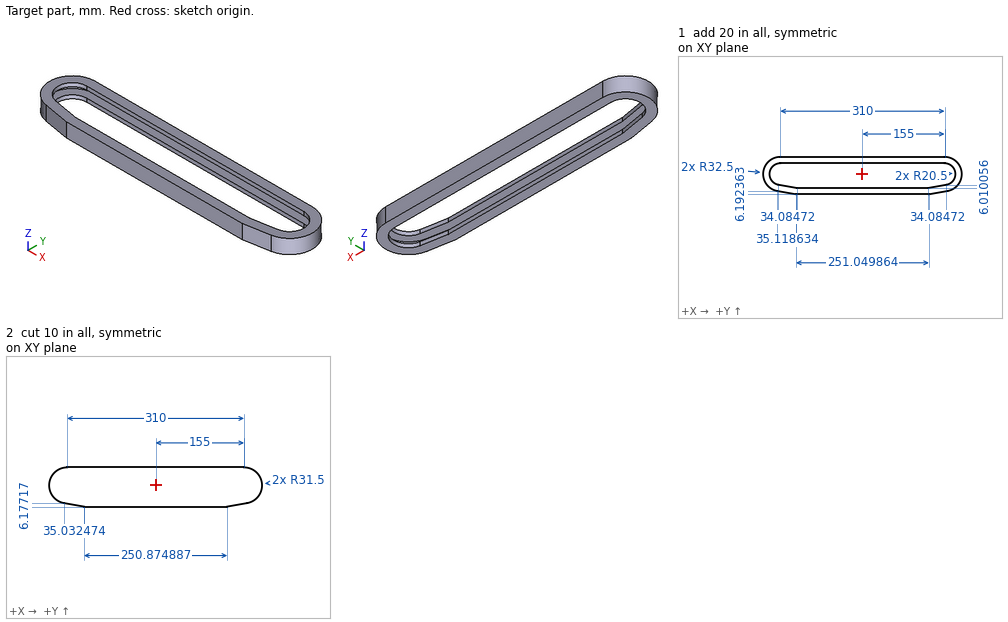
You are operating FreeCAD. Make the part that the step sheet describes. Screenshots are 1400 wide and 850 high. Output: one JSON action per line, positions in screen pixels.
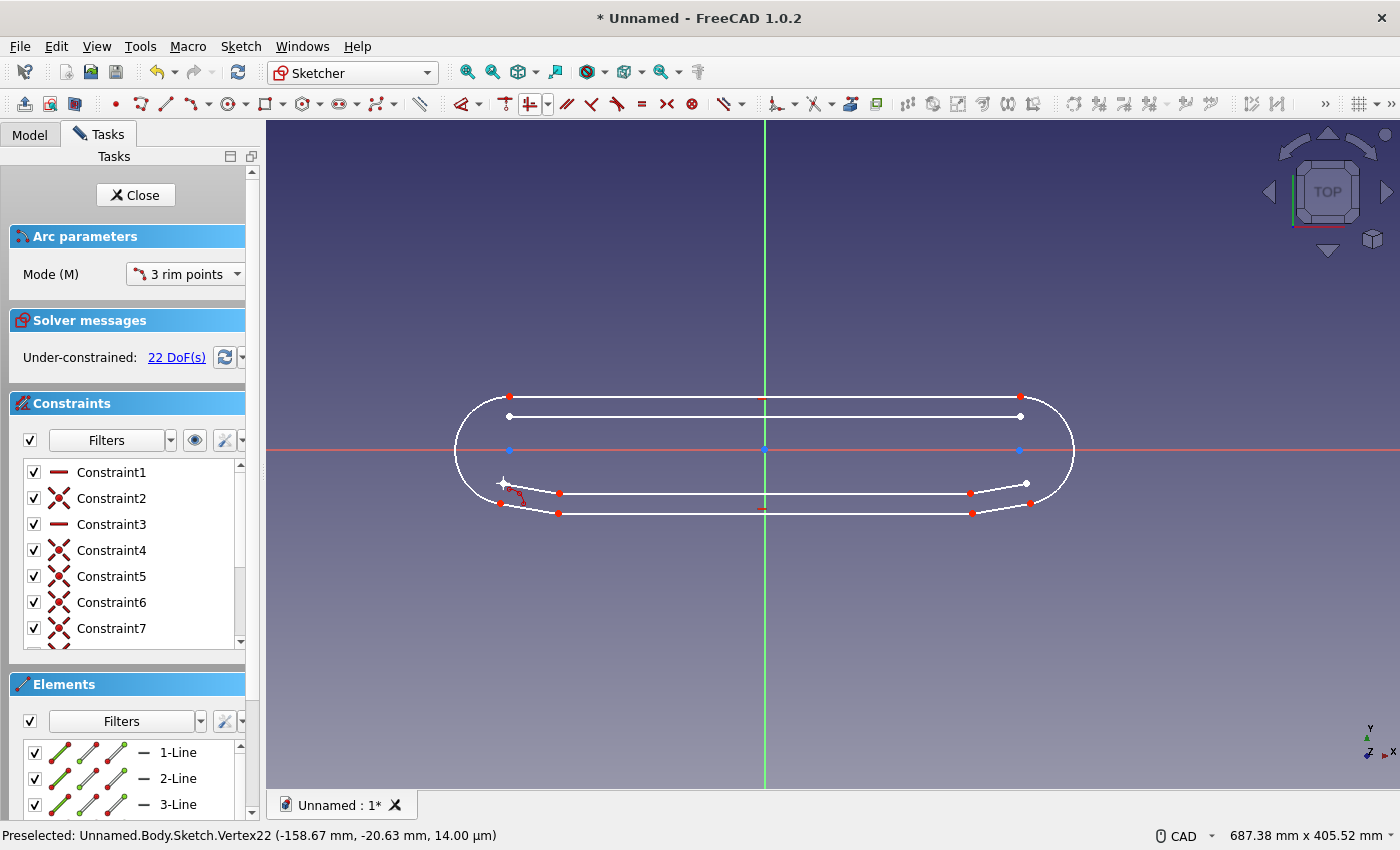
{"action": "left_click", "coordinate": [1020, 417]}
{"action": "left_click", "coordinate": [1026, 484]}
{"action": "left_click", "coordinate": [1050, 466]}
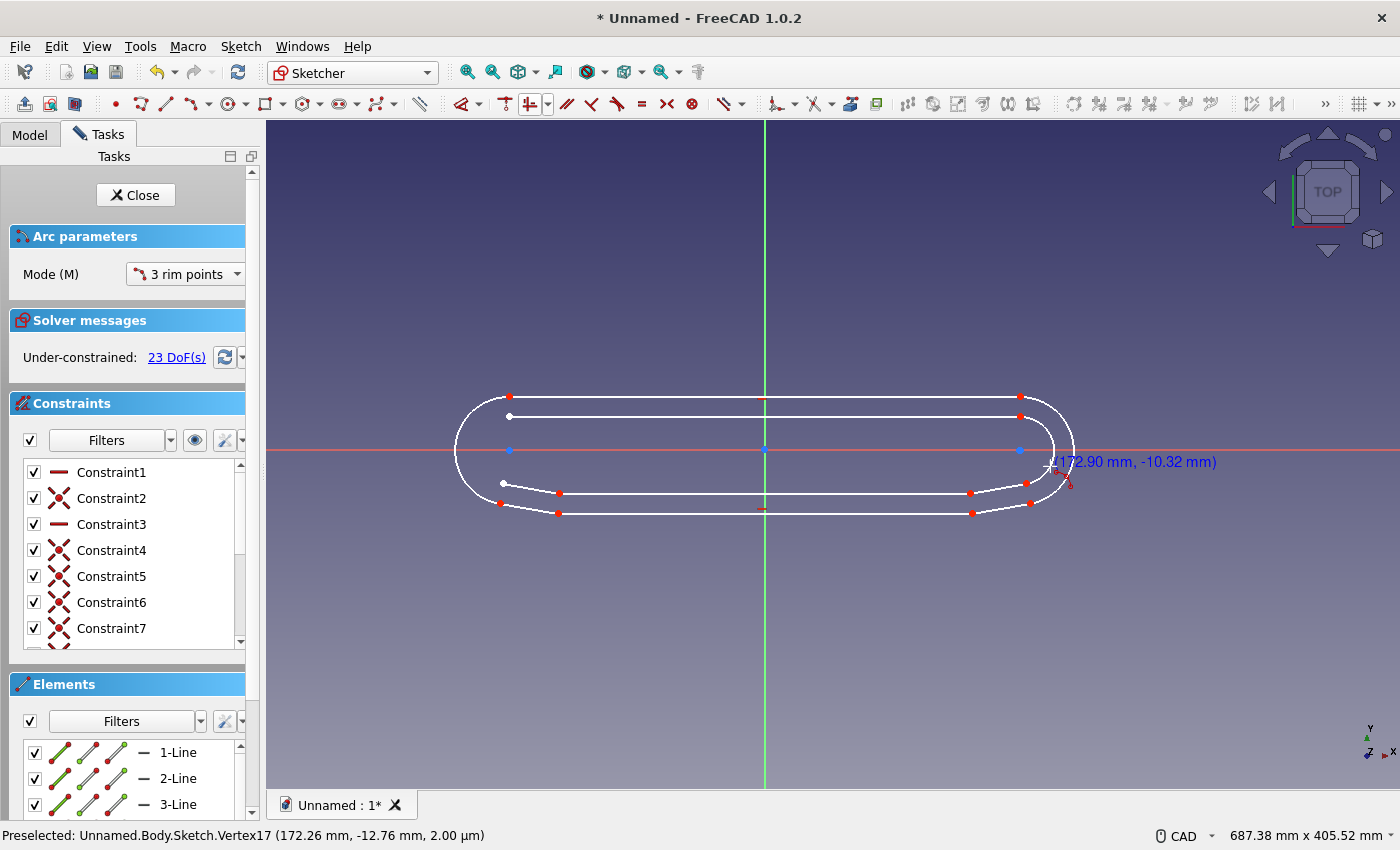
{"action": "left_click", "coordinate": [503, 484]}
{"action": "left_click", "coordinate": [509, 417]}
{"action": "left_click", "coordinate": [483, 429]}
{"action": "key", "text": "Escape"}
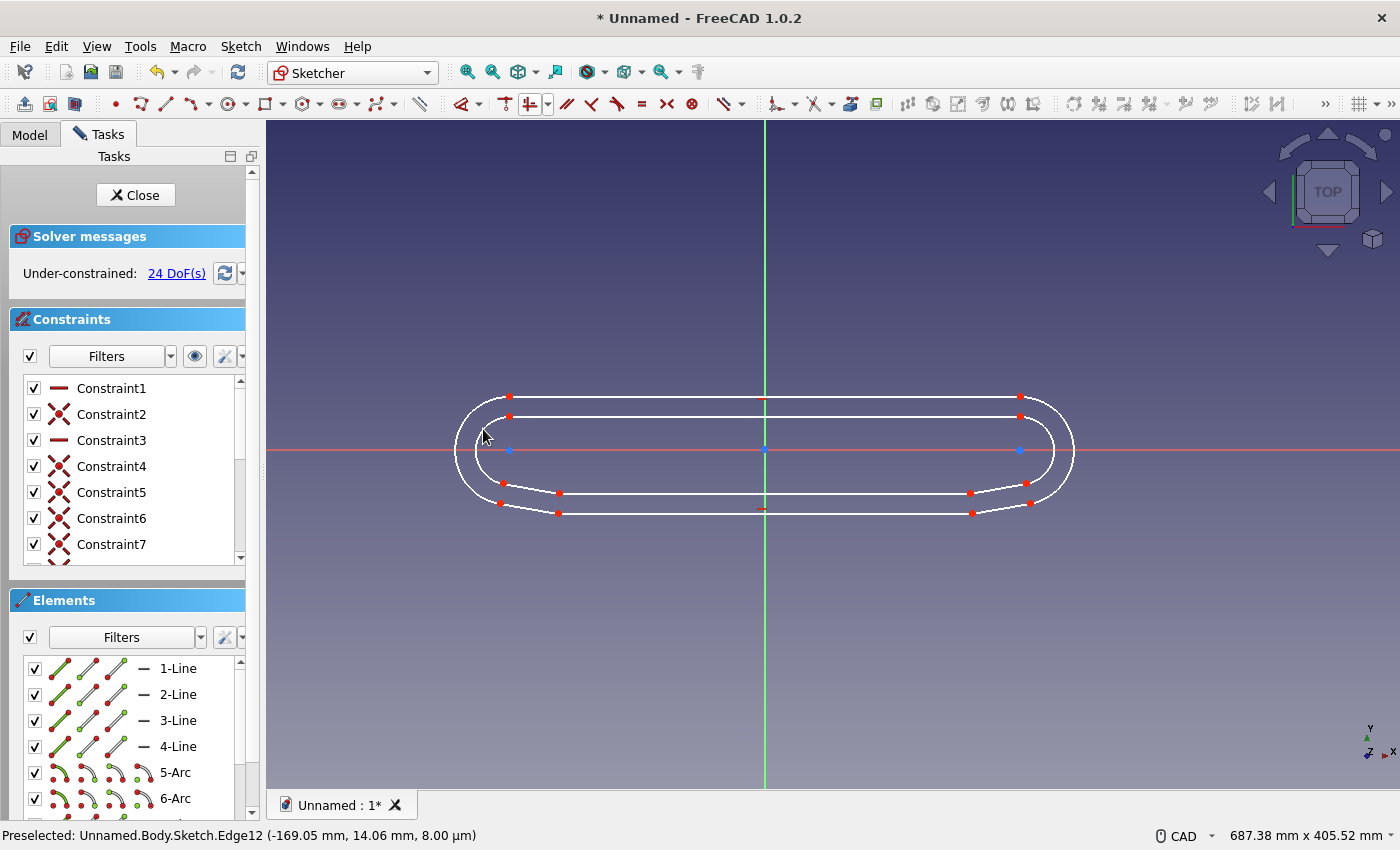
{"action": "left_click", "coordinate": [867, 397]}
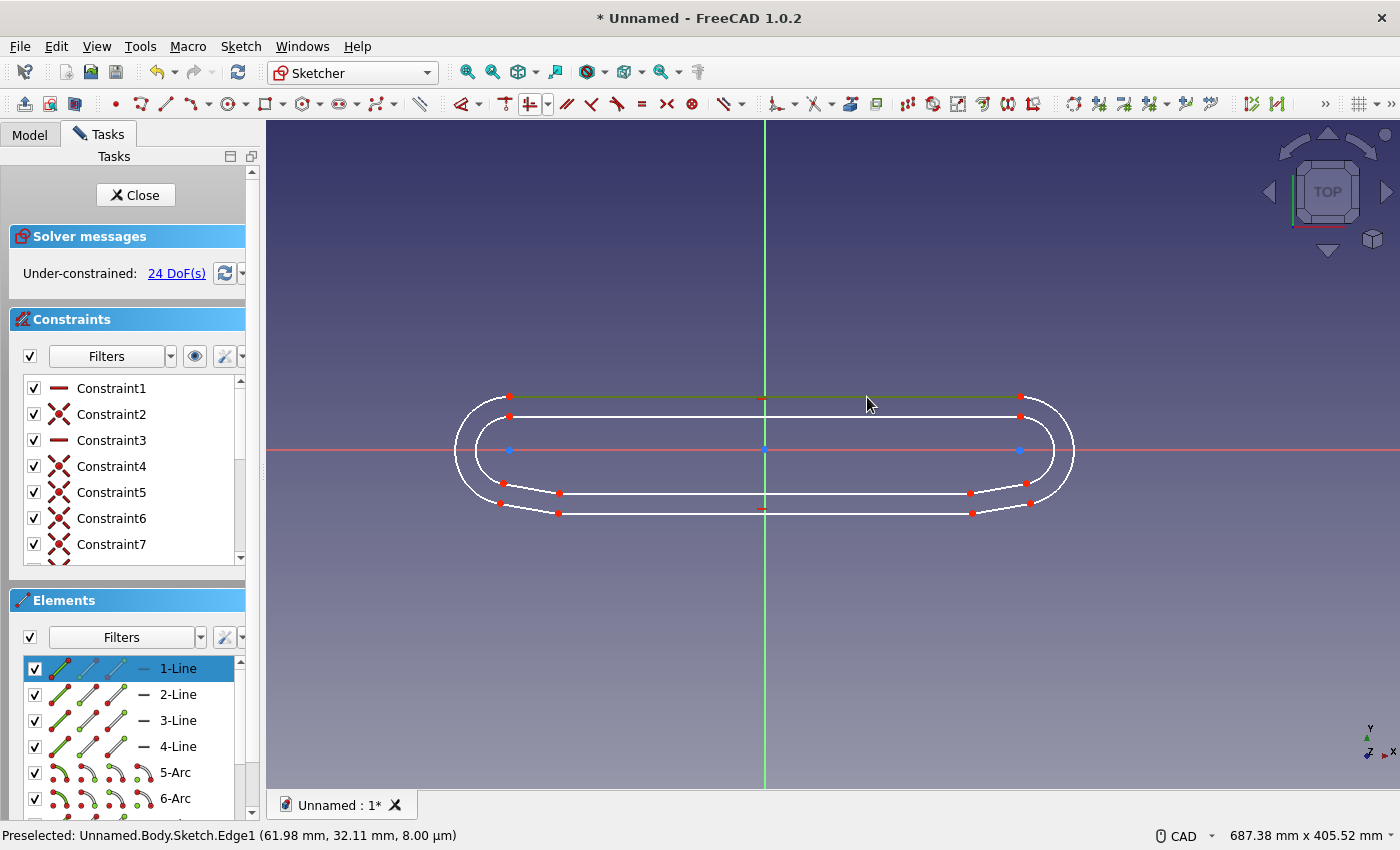
{"action": "left_click", "coordinate": [467, 417]}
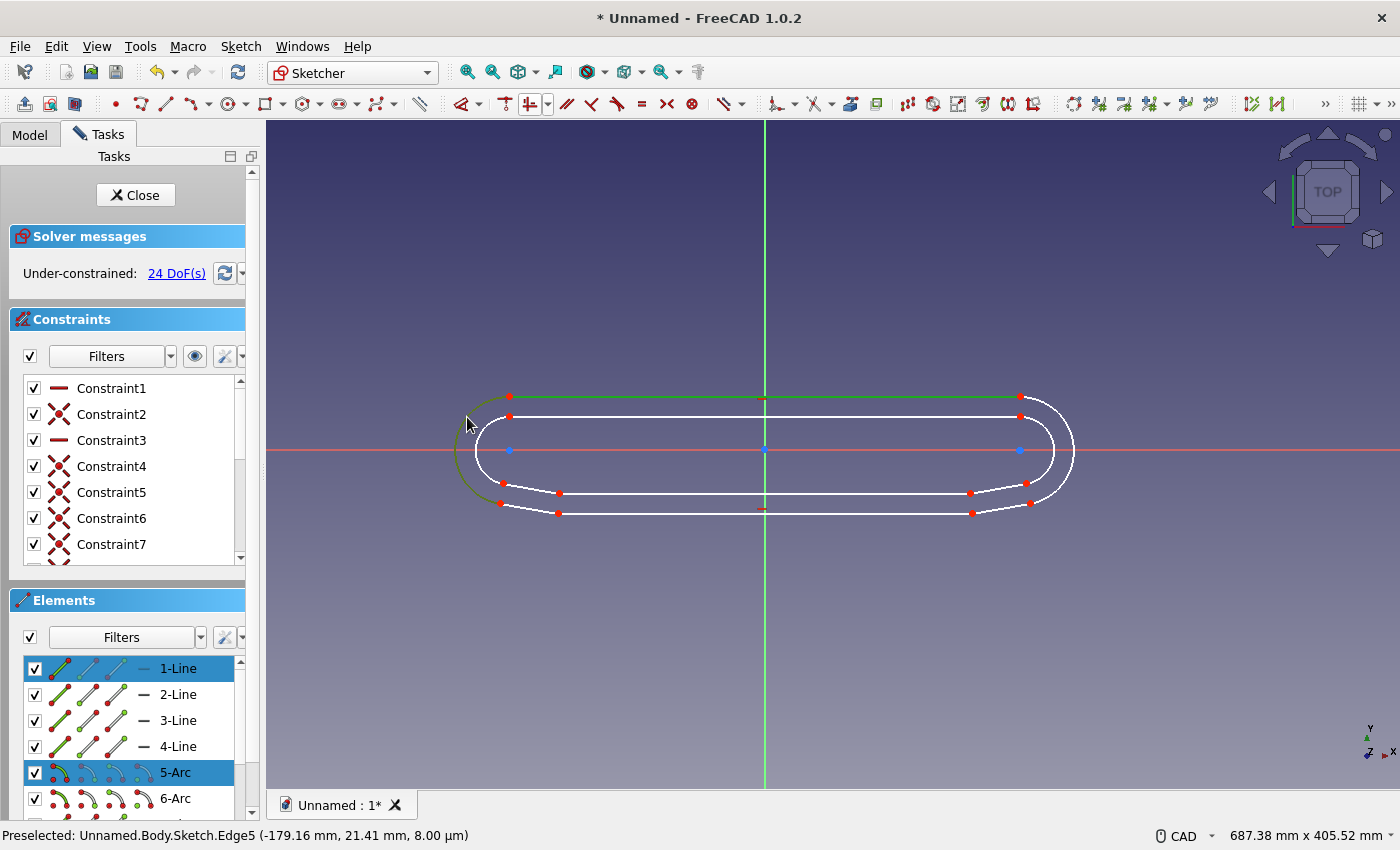
{"action": "key", "text": "t"}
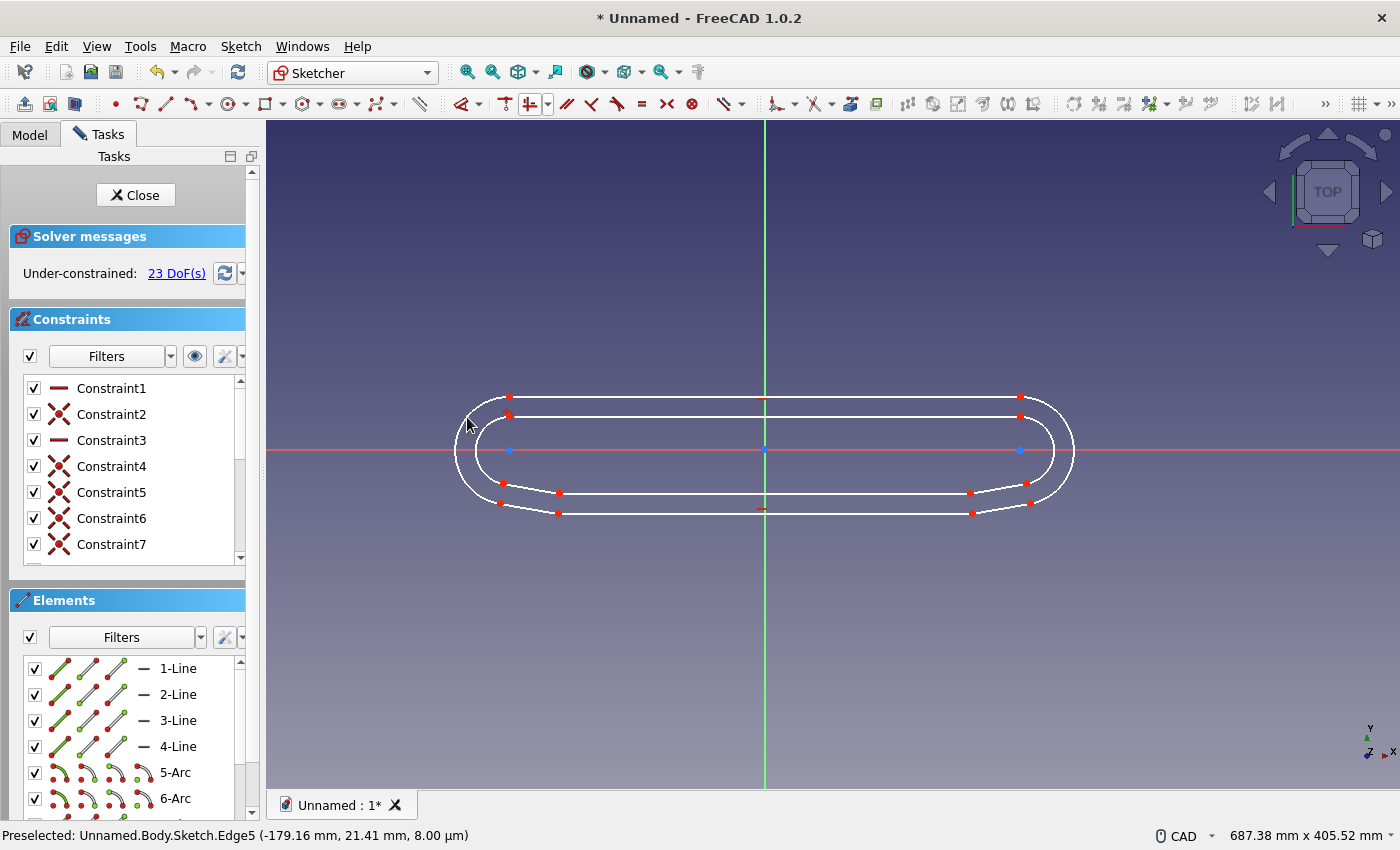
{"action": "left_click", "coordinate": [867, 397]}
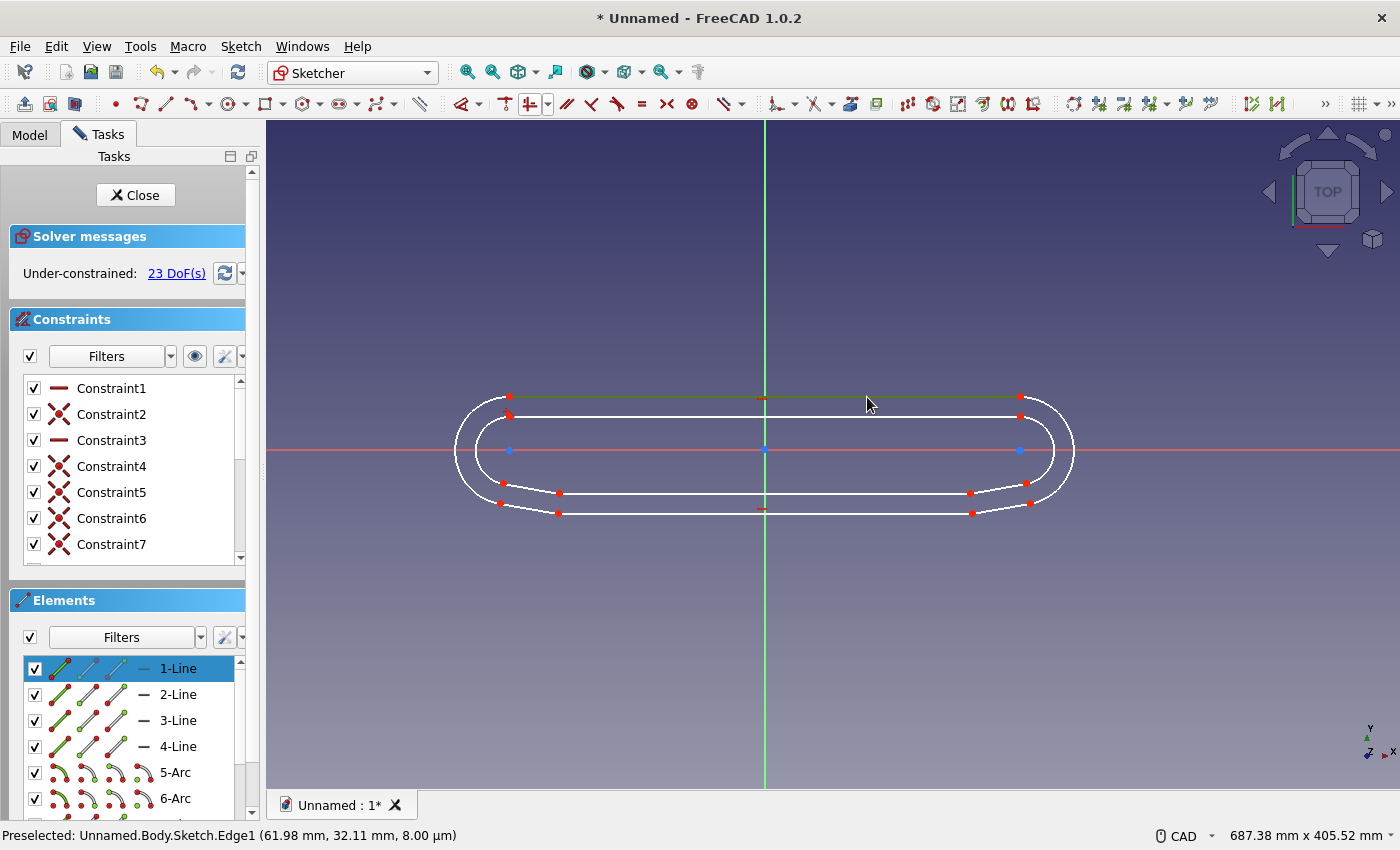
{"action": "left_click", "coordinate": [1067, 477]}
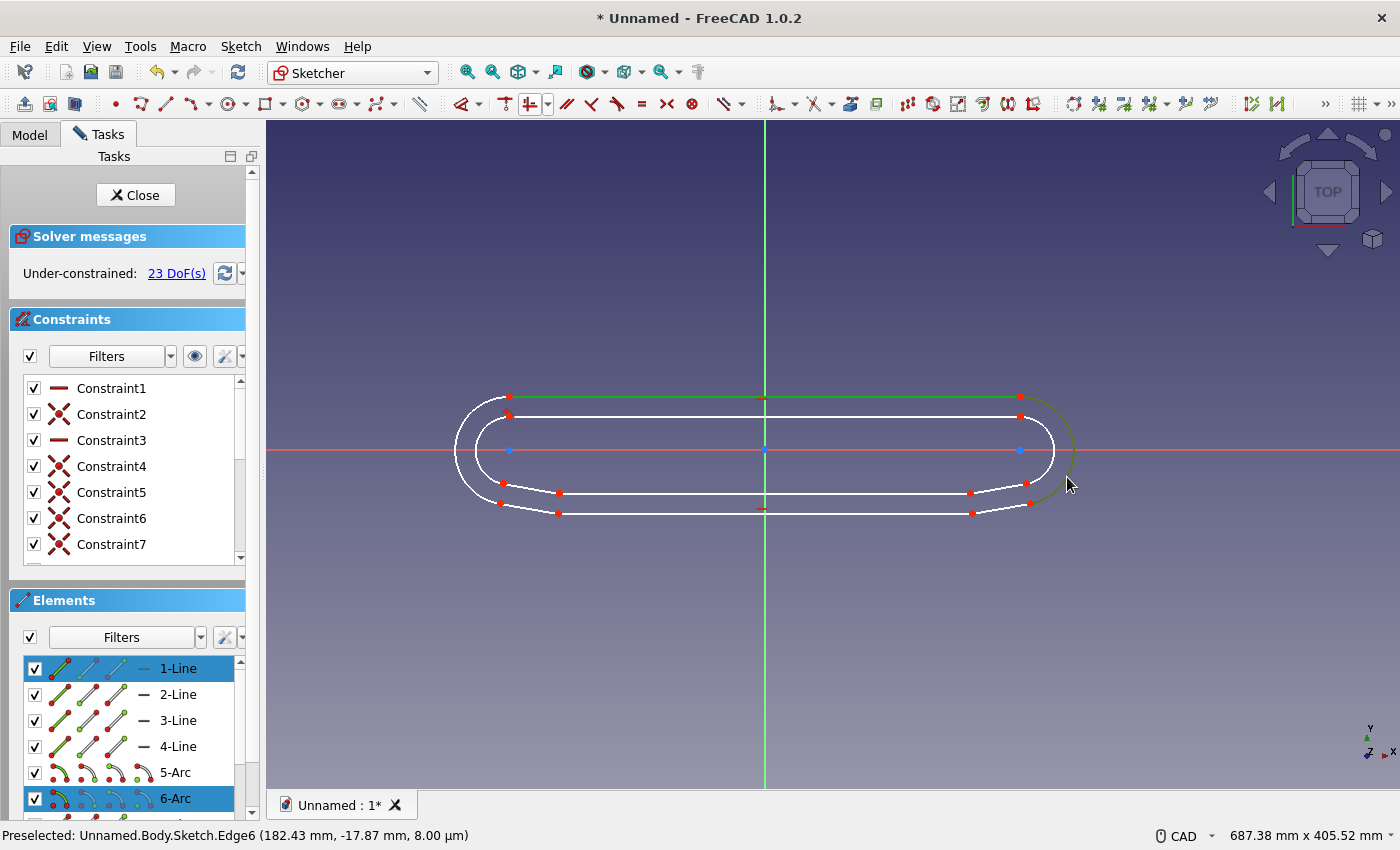
{"action": "left_click", "coordinate": [617, 104]}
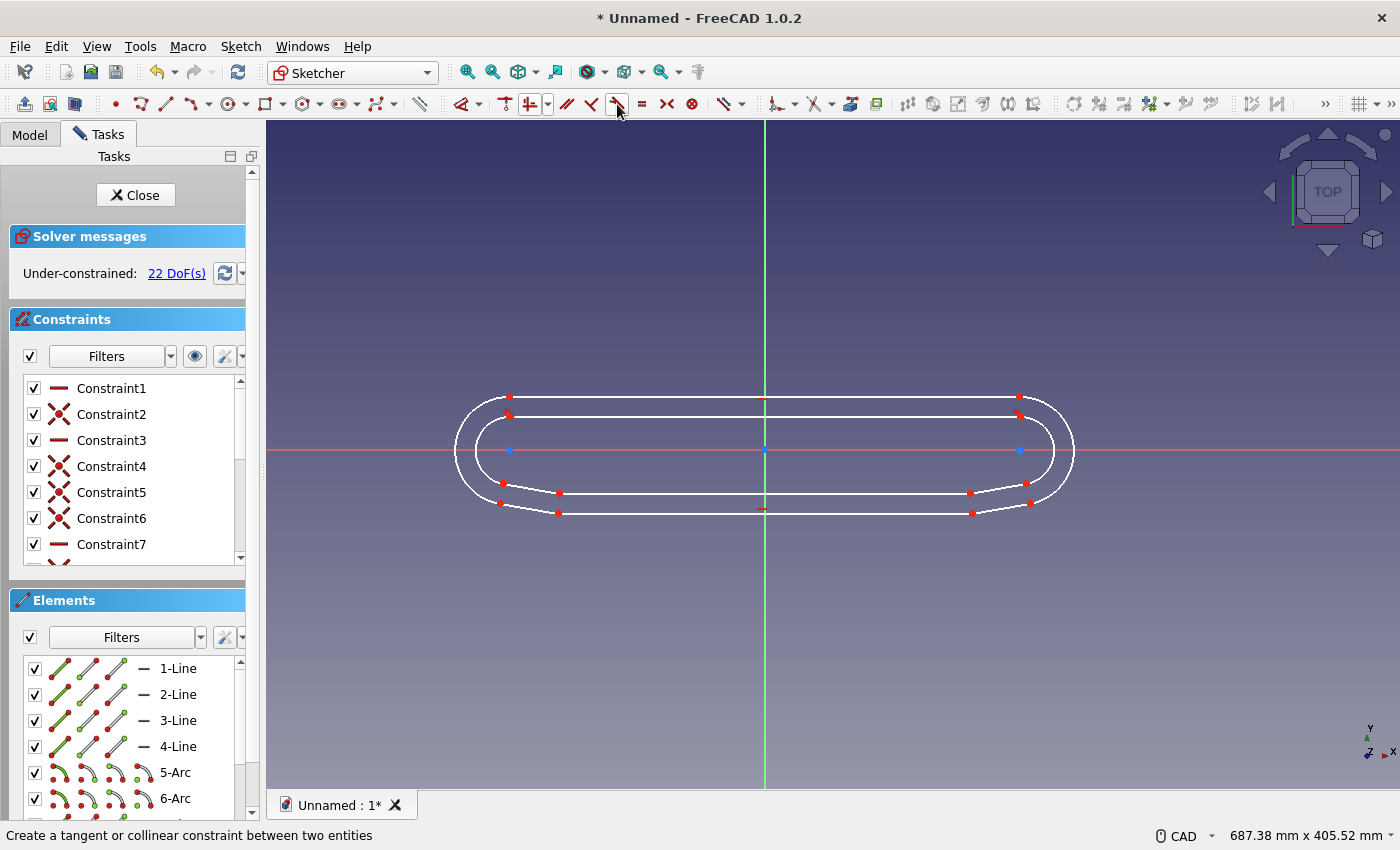
{"action": "left_click", "coordinate": [517, 507]}